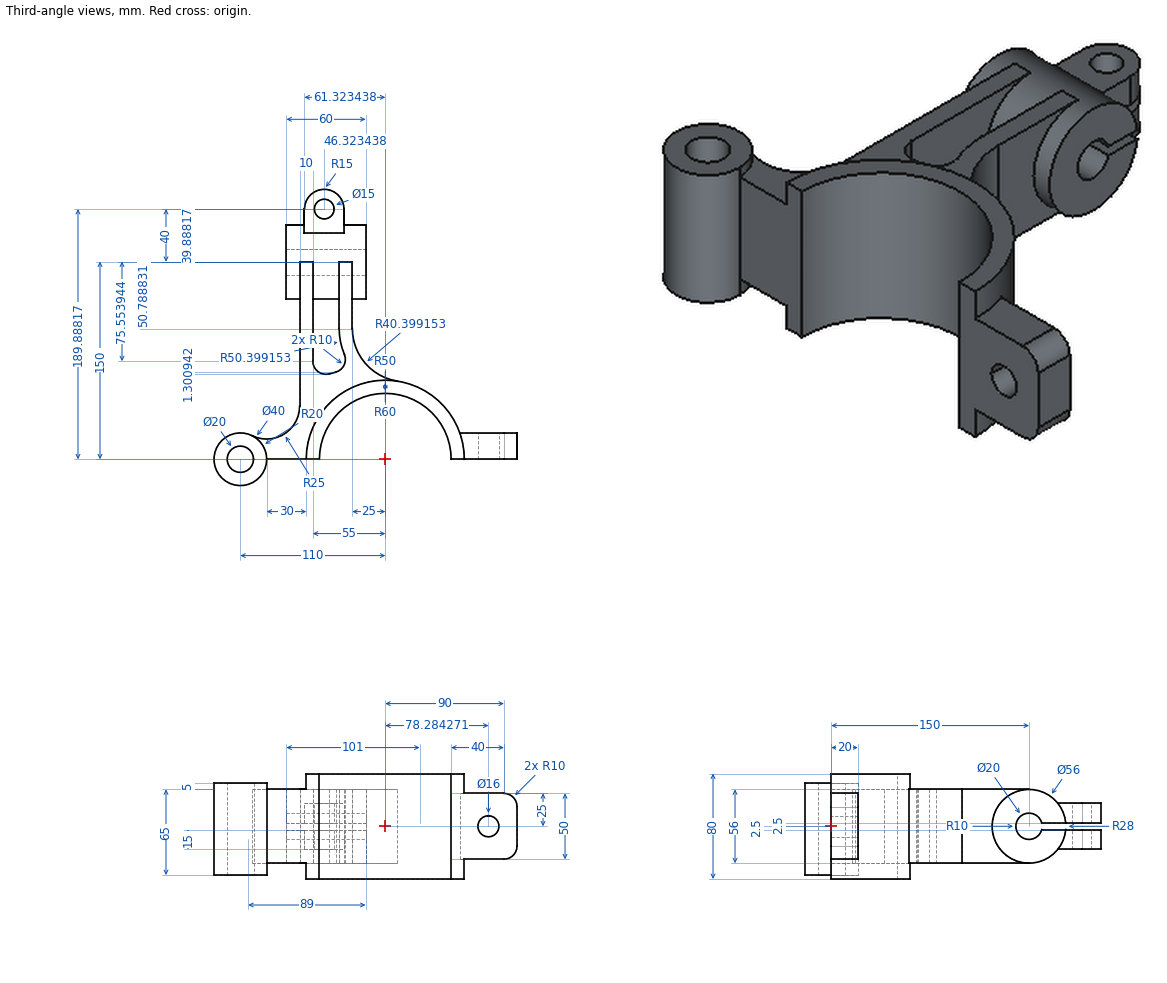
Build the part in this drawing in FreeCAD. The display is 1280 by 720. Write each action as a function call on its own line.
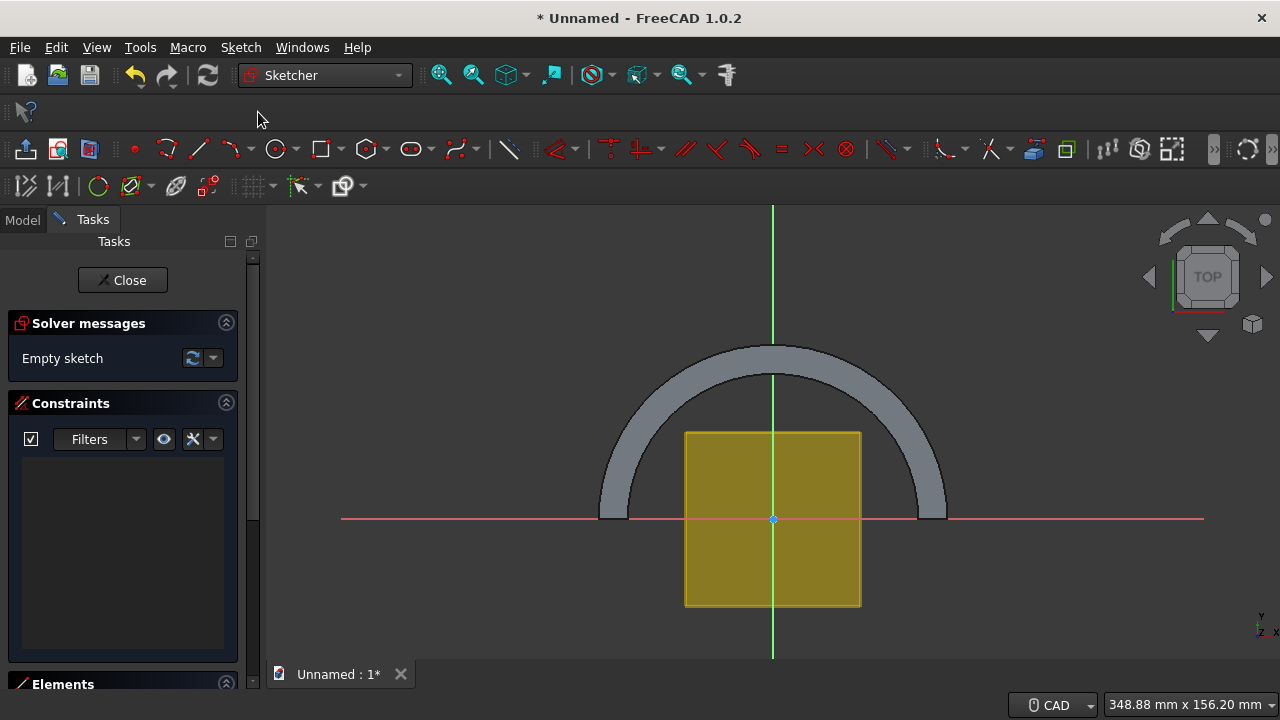
scroll(294, 590, up, 4)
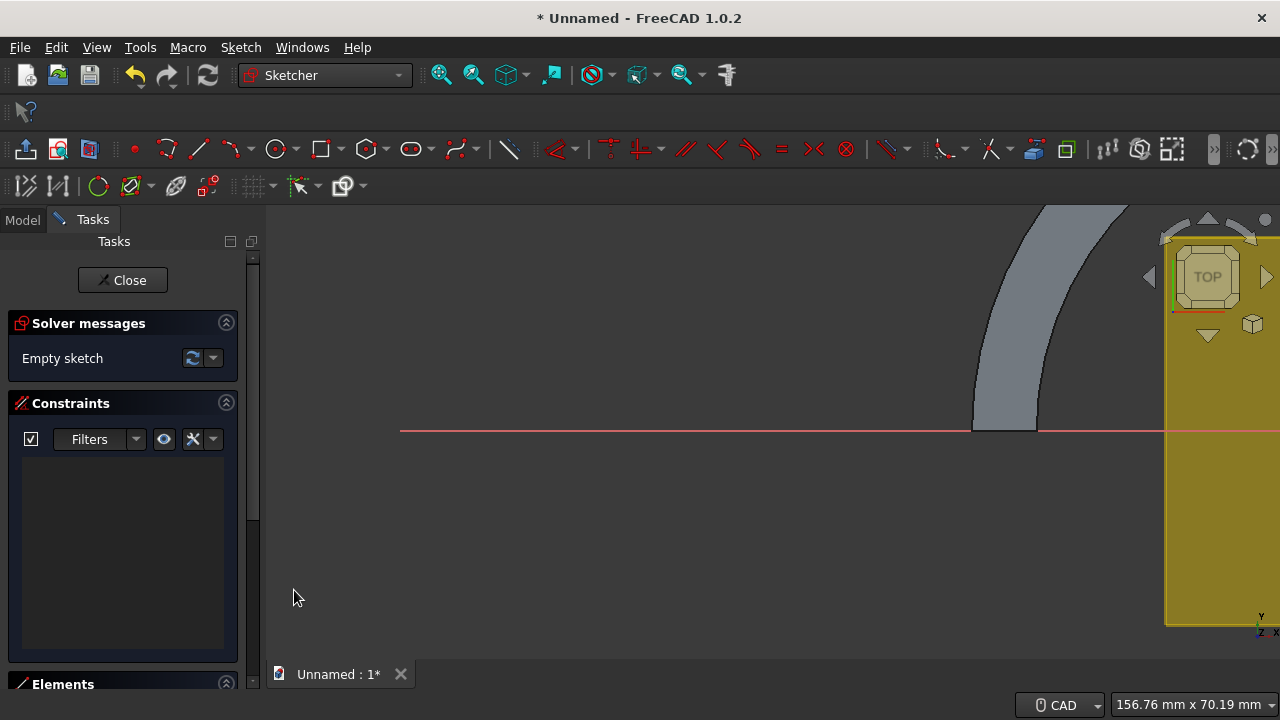
click(276, 150)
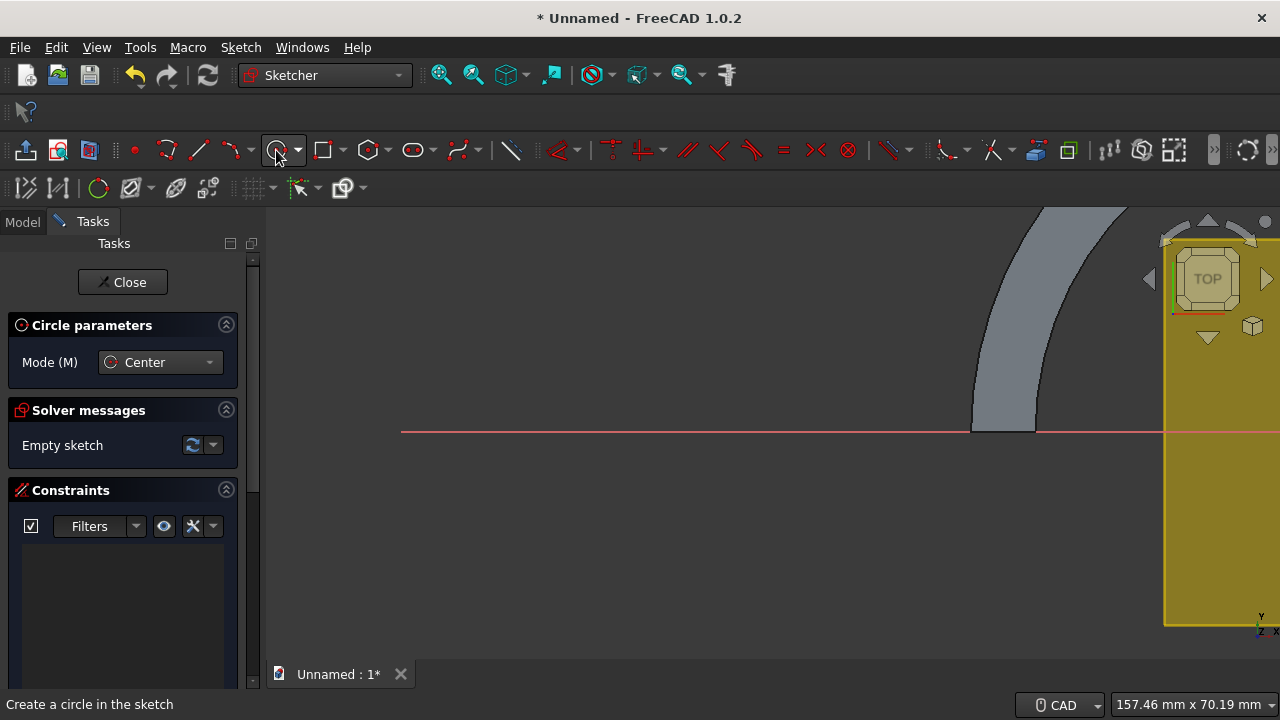
click(649, 432)
move(740, 341)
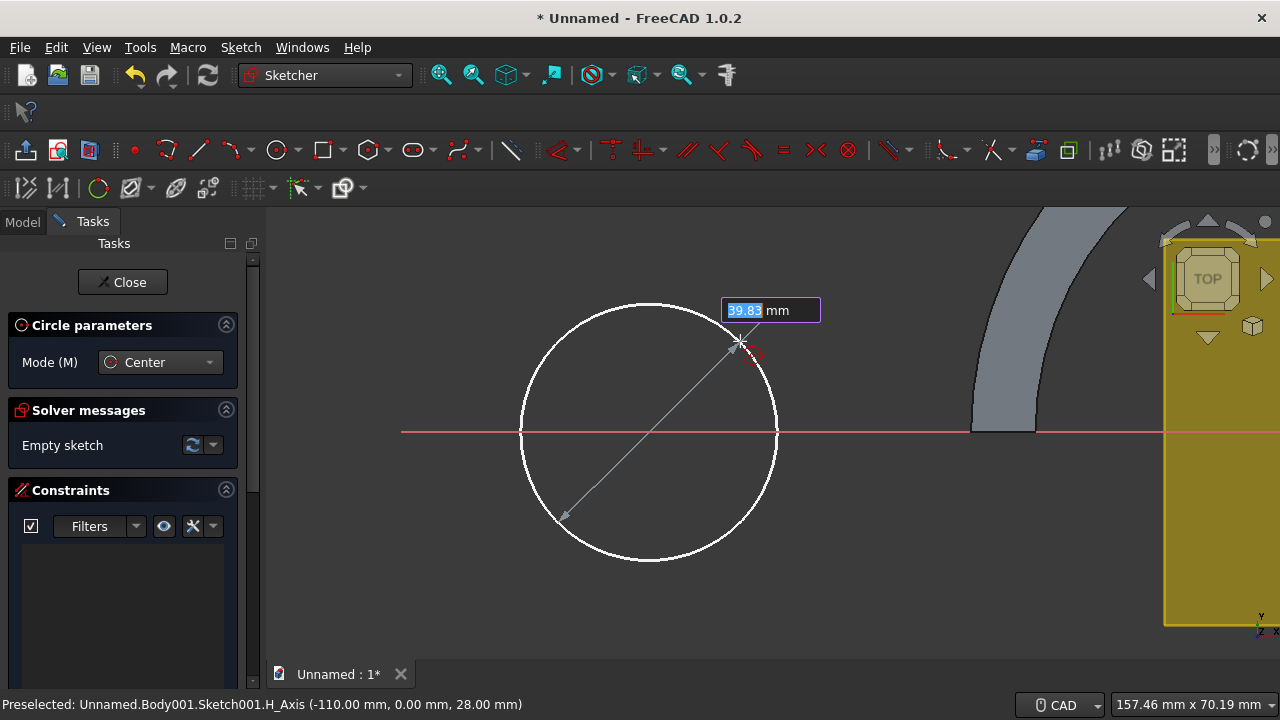
text(40)
key(Return)
key(Escape)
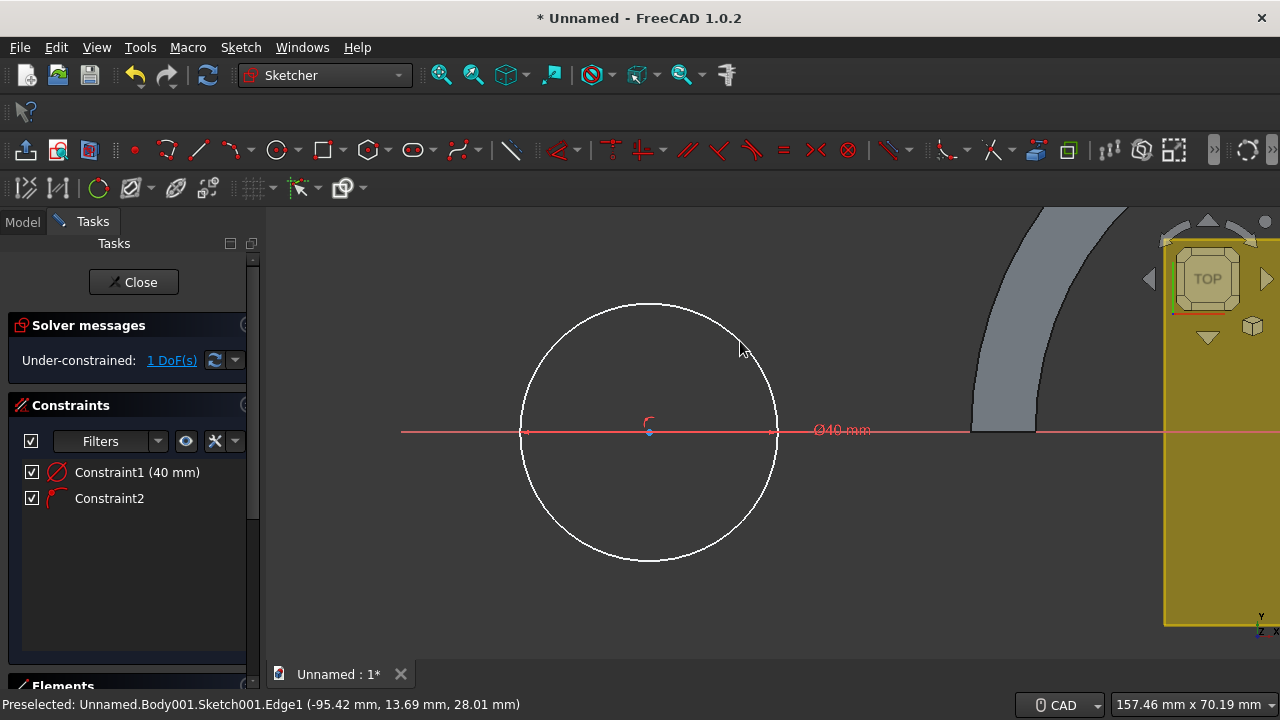
key(d)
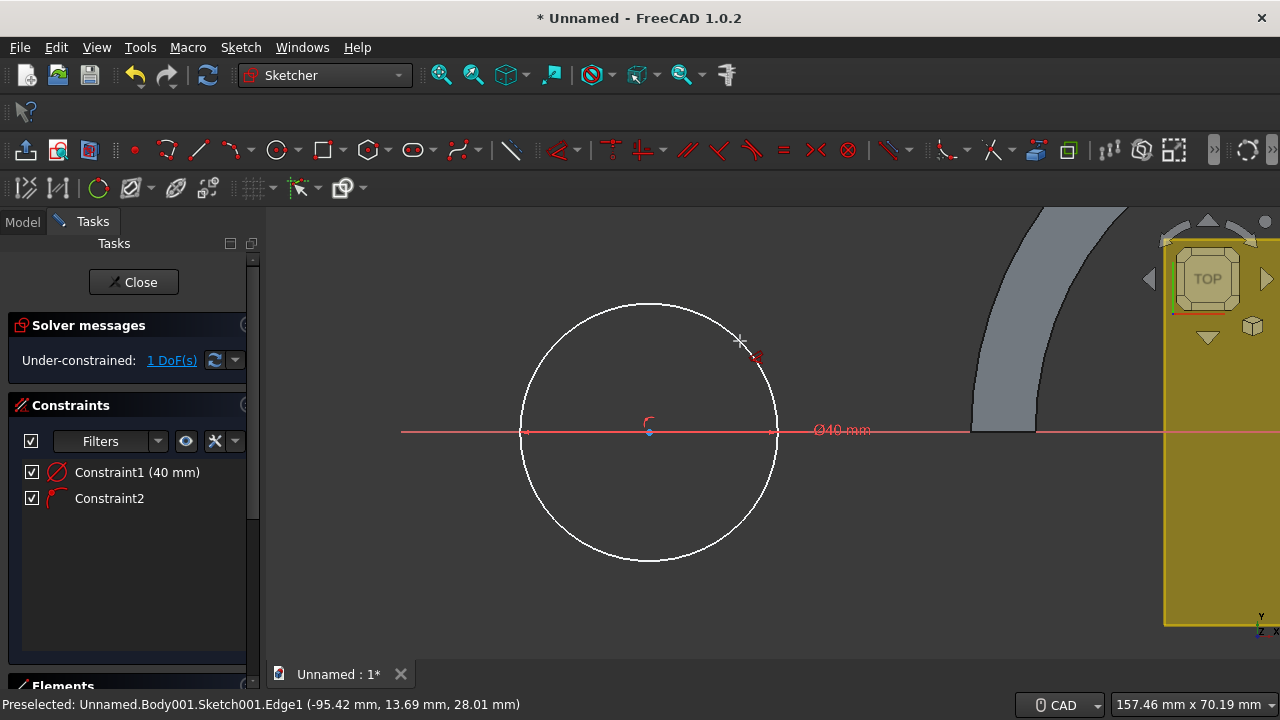
click(649, 432)
click(882, 466)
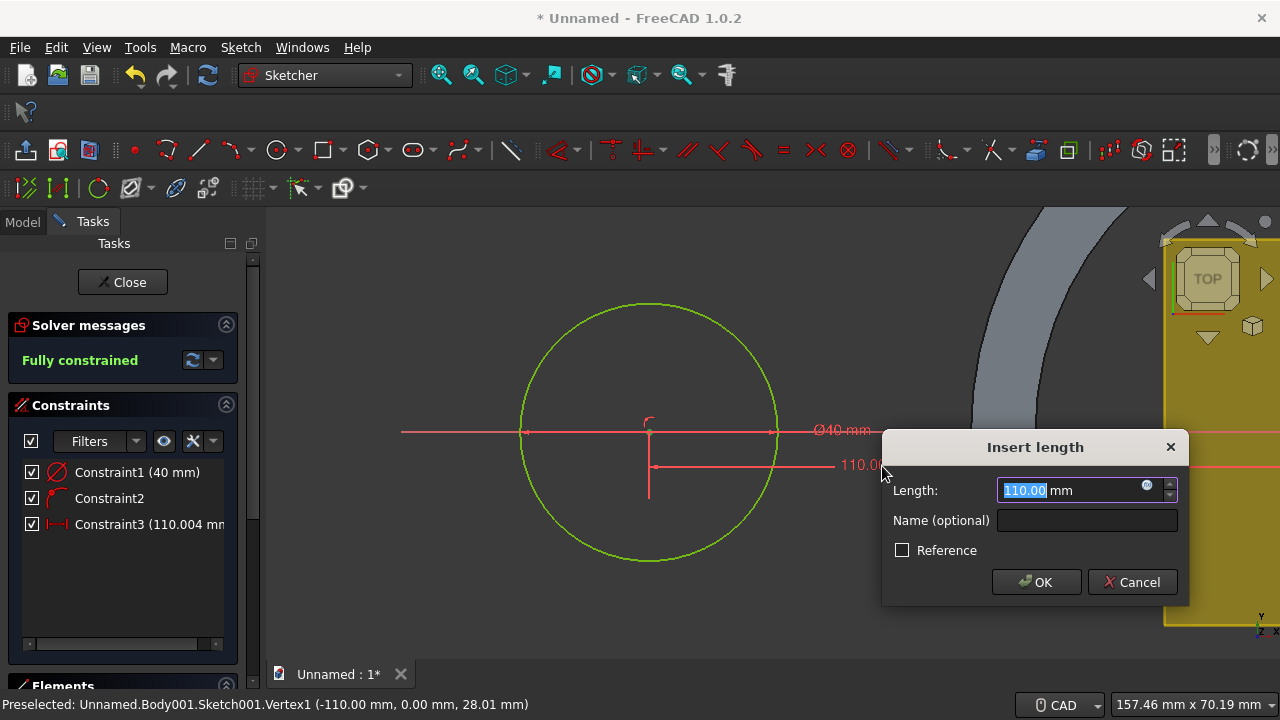
text(110)
key(Return)
key(Escape)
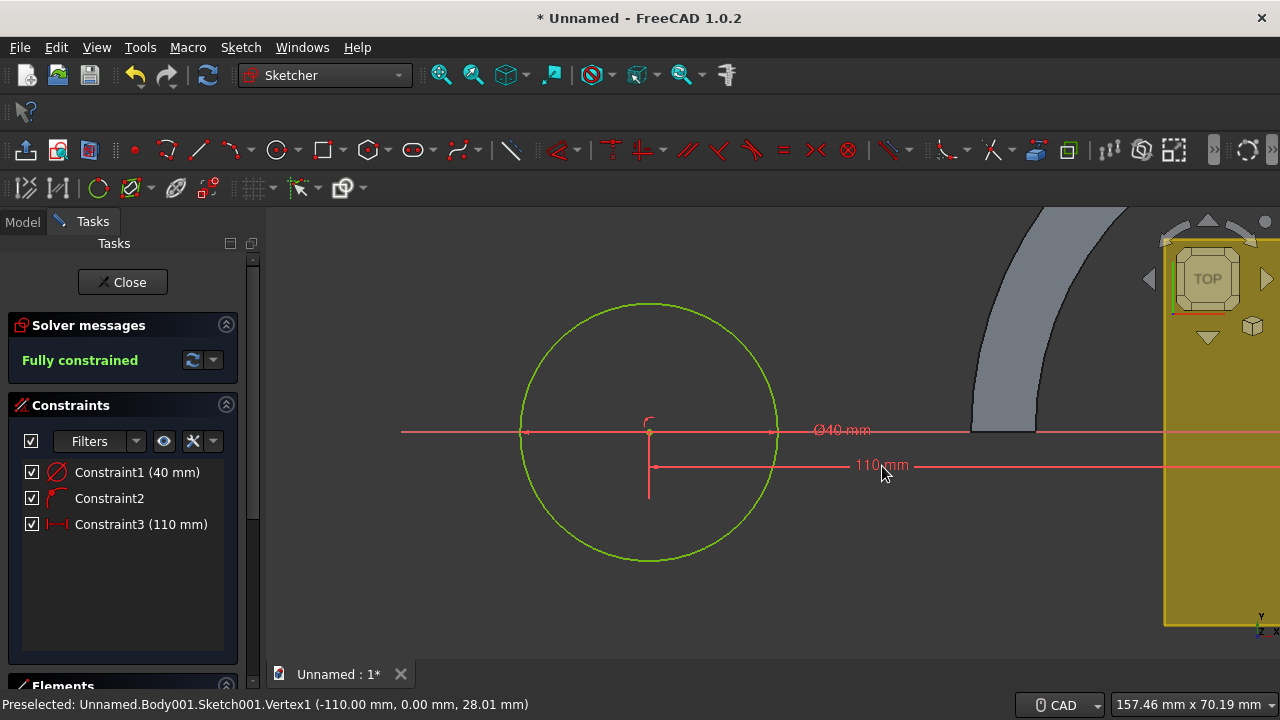
click(123, 282)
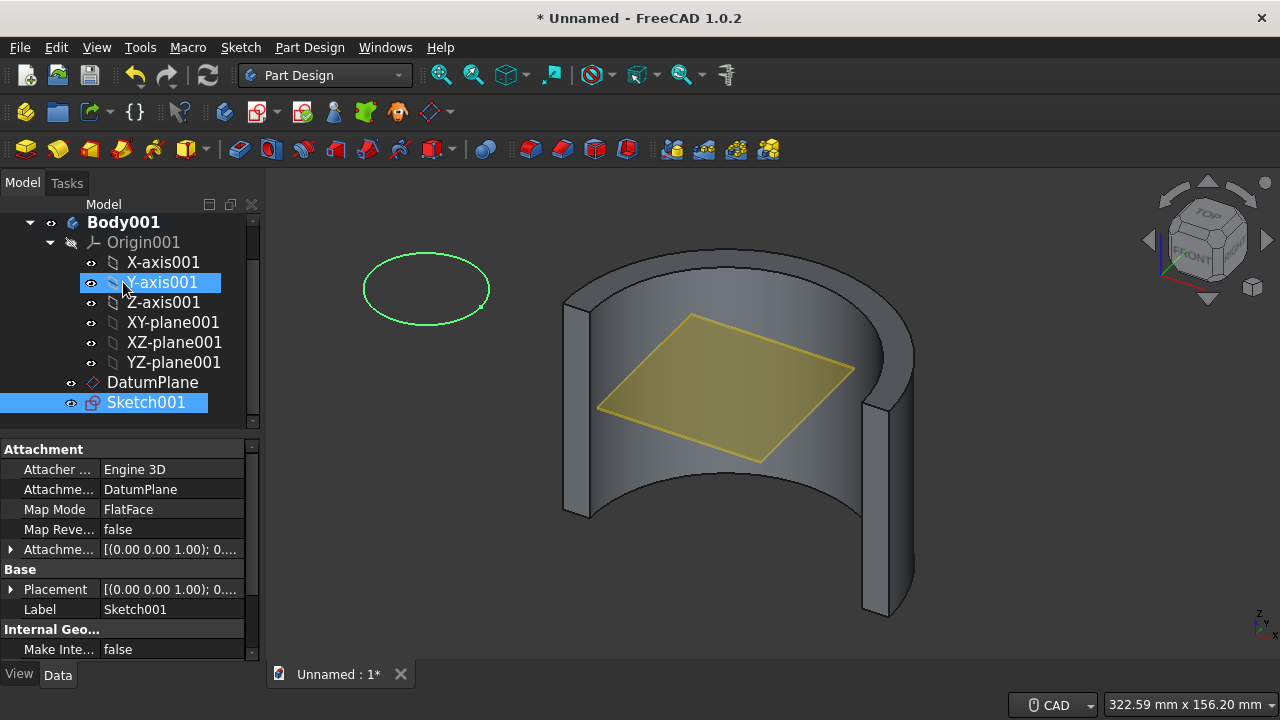
click(26, 150)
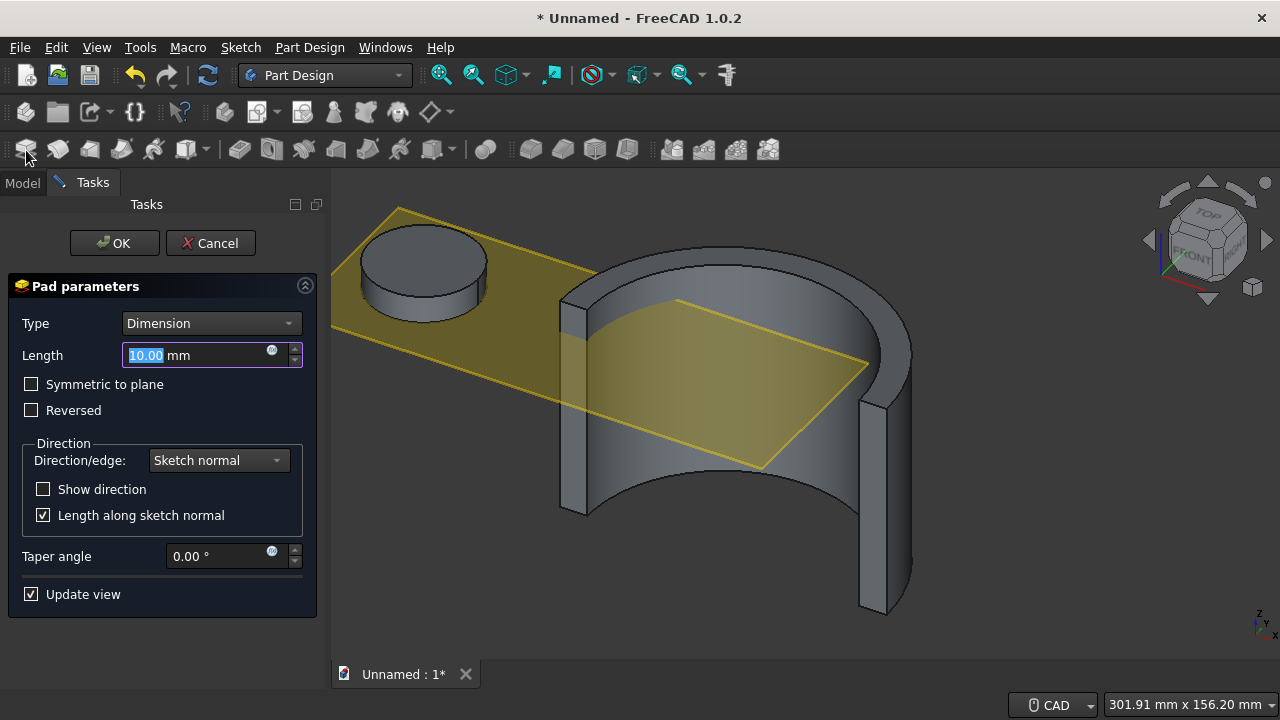
click(212, 324)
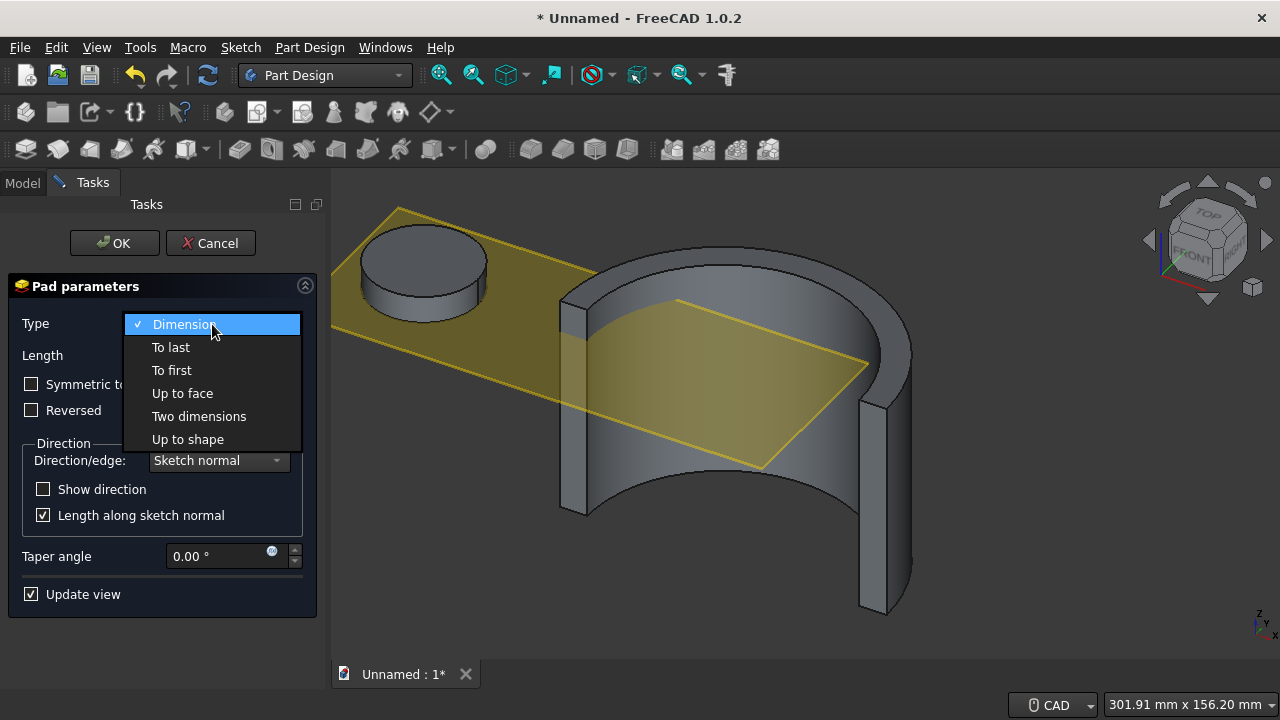
click(212, 416)